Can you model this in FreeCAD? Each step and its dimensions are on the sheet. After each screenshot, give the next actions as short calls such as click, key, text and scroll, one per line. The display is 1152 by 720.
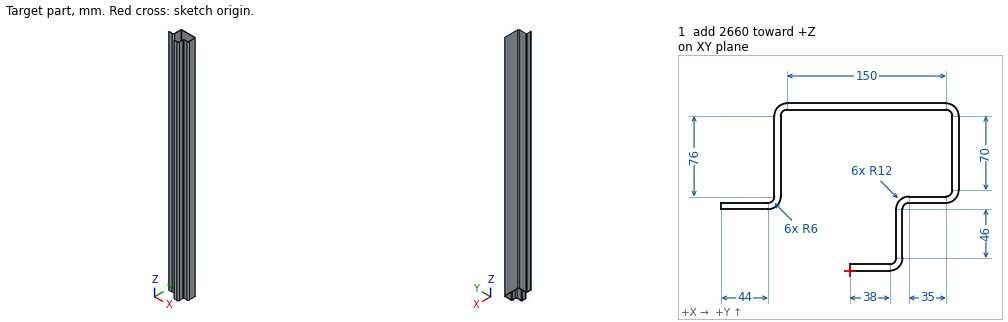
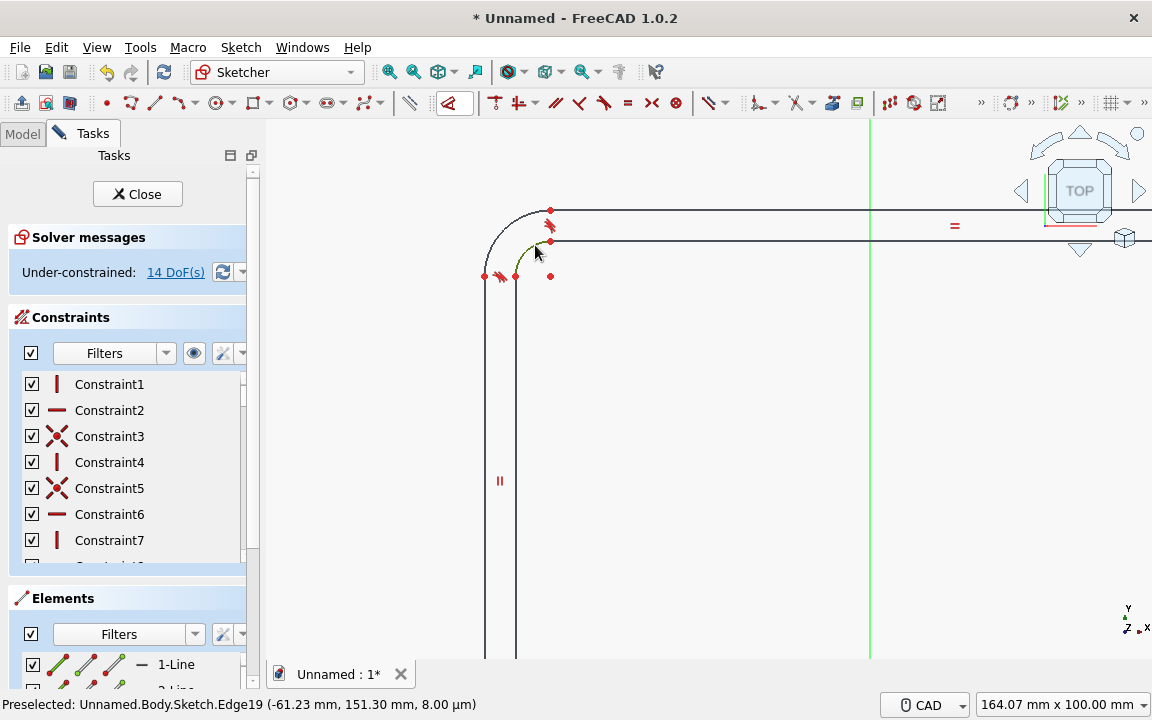
scroll(535, 246, down, 5)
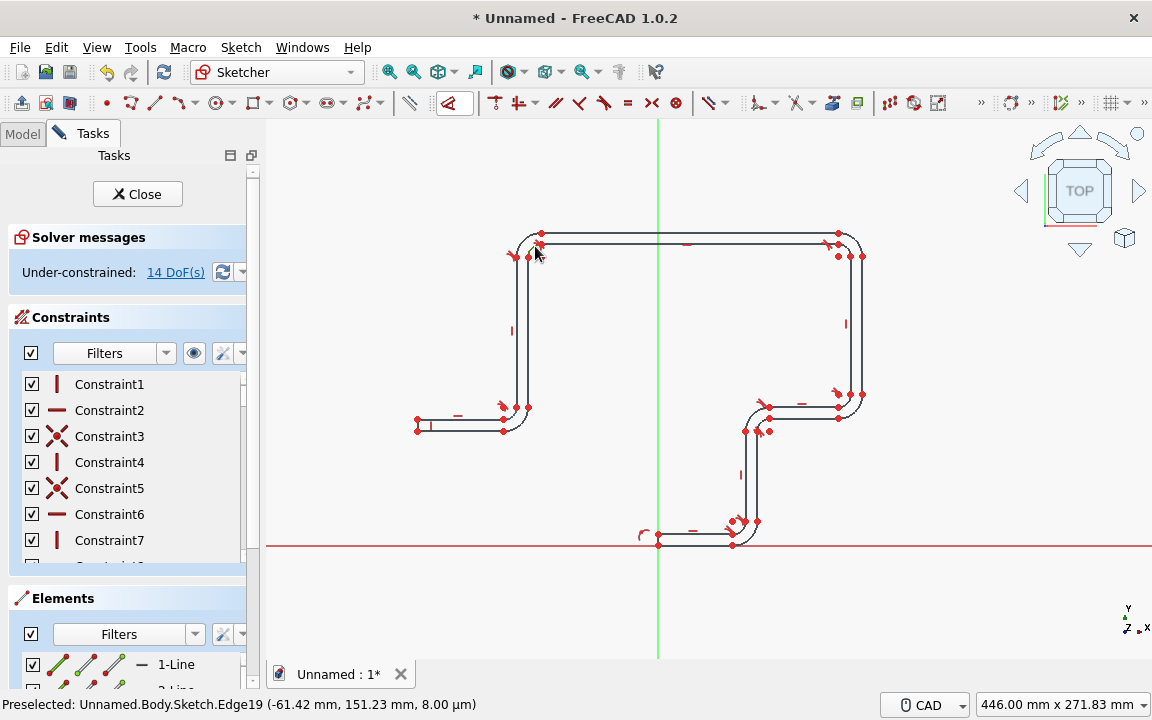
scroll(850, 251, up, 5)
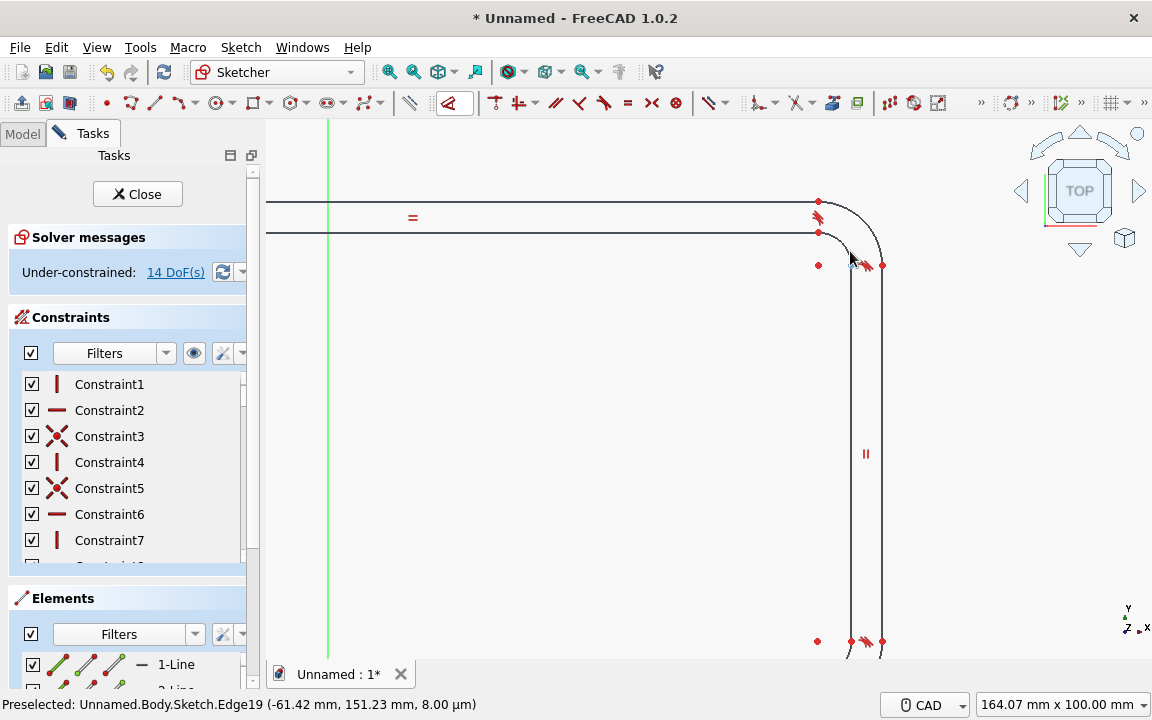
click(848, 251)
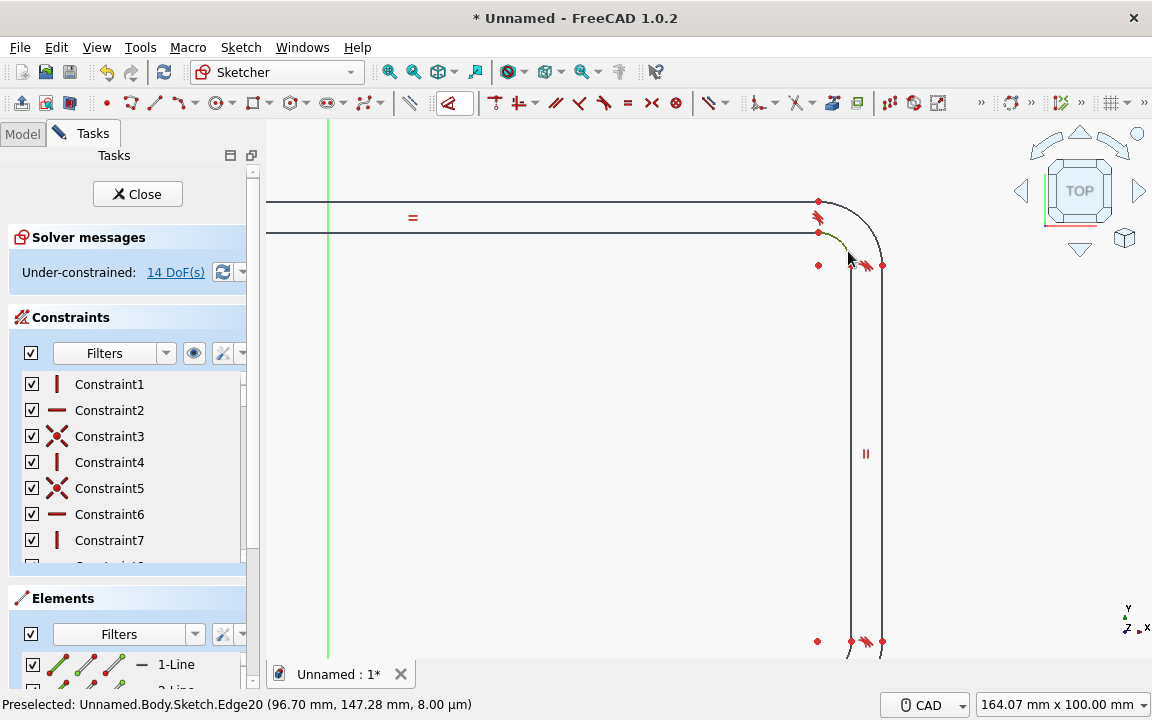
scroll(851, 251, down, 5)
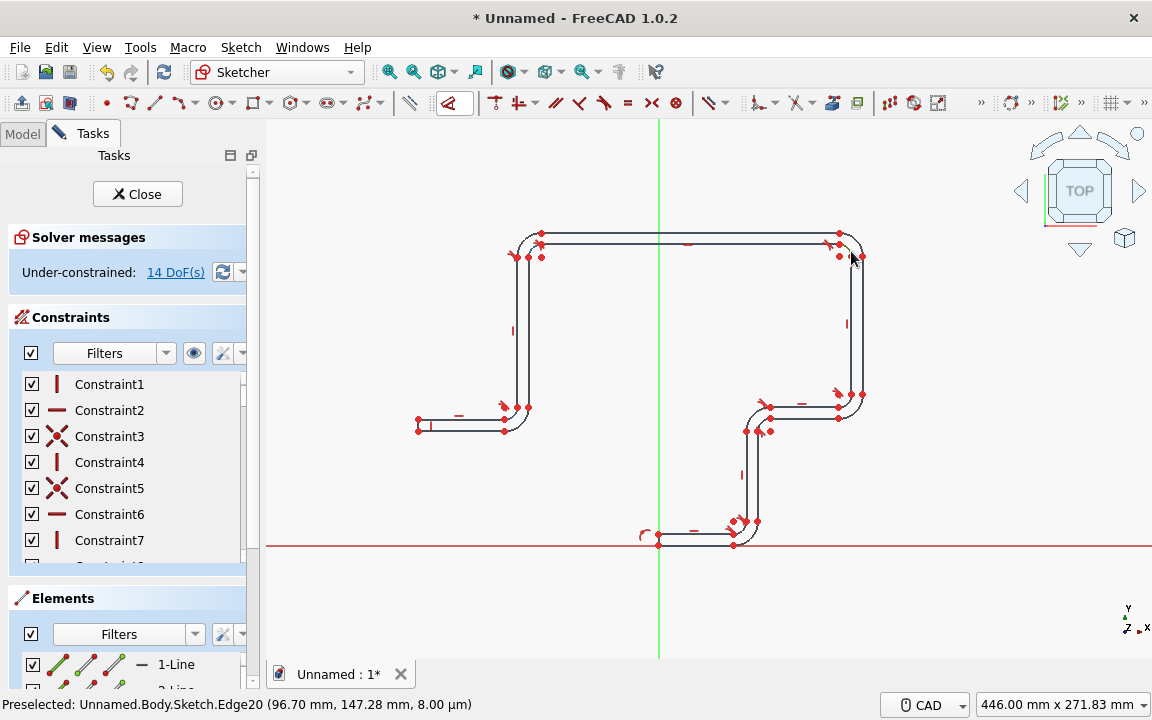
scroll(845, 406, up, 5)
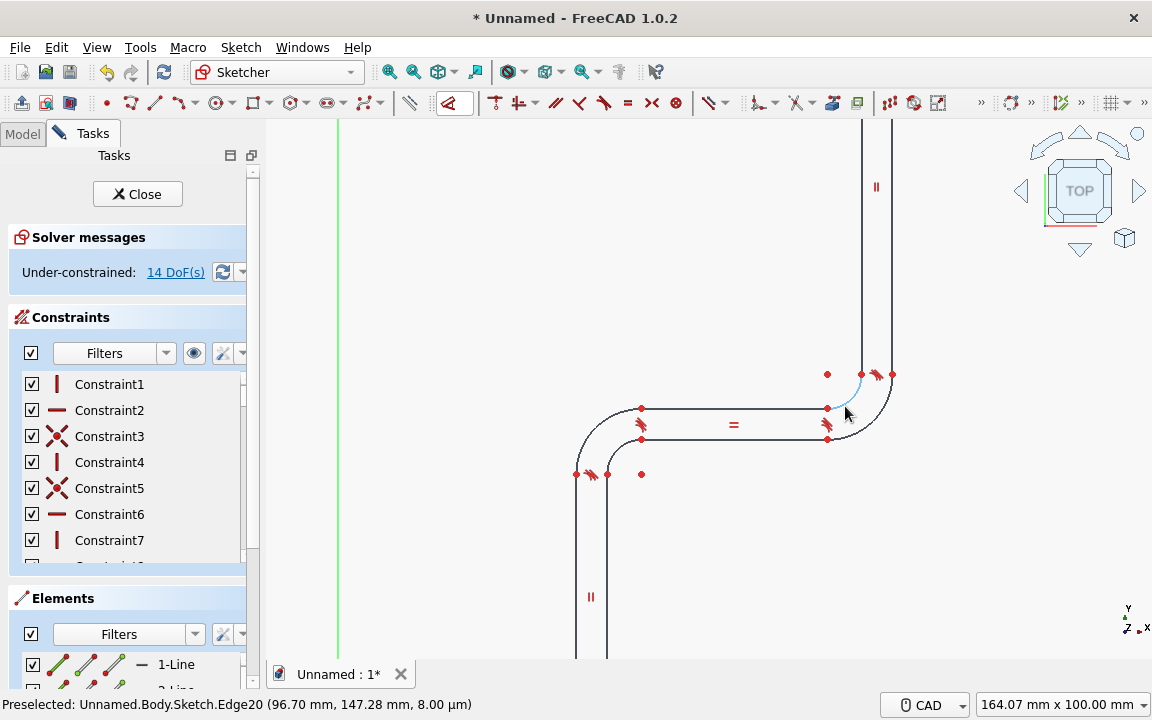
click(843, 405)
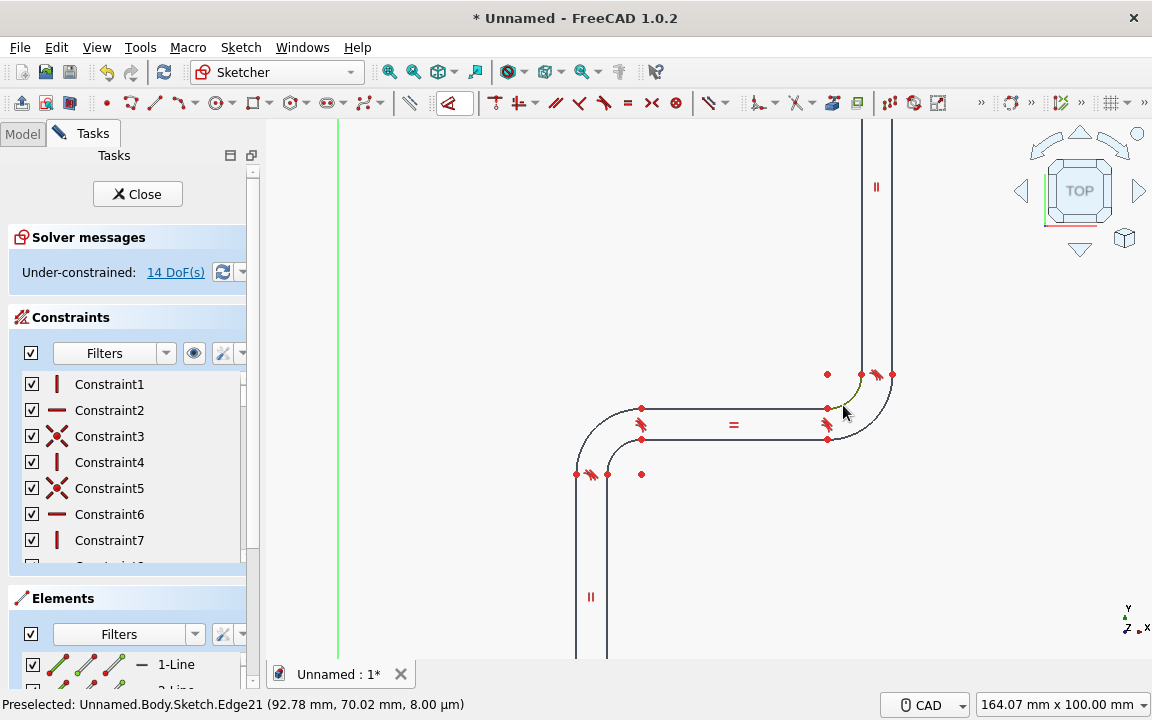
scroll(845, 407, down, 5)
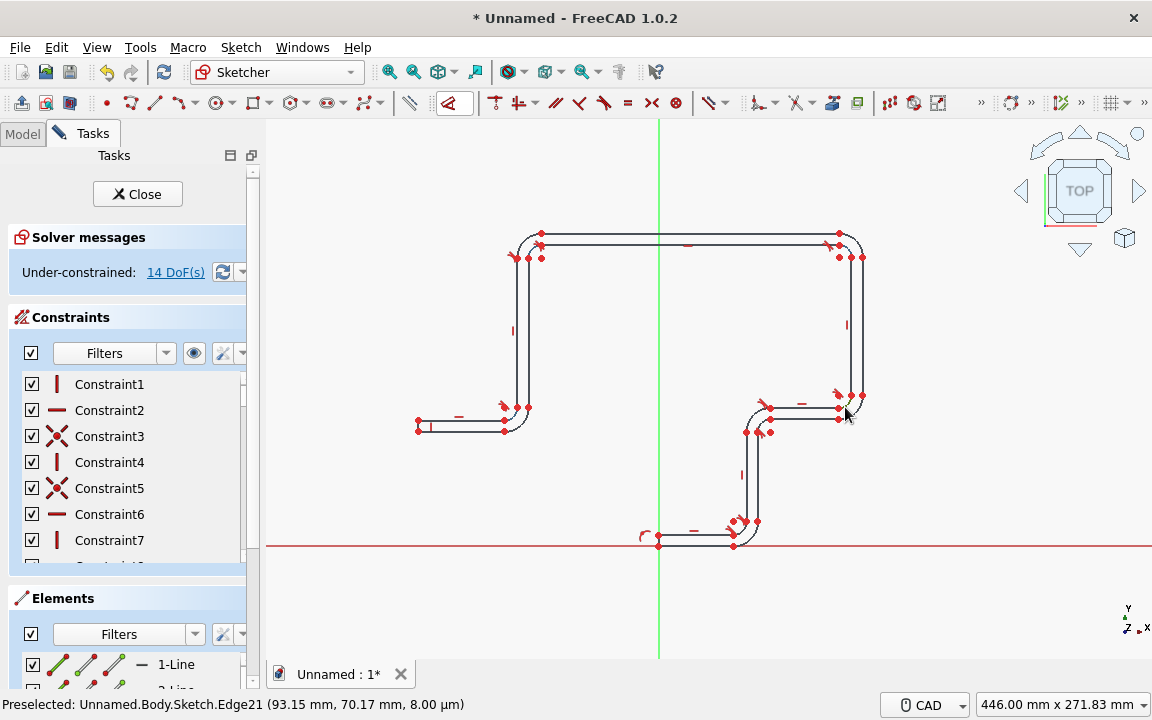
scroll(739, 534, up, 4)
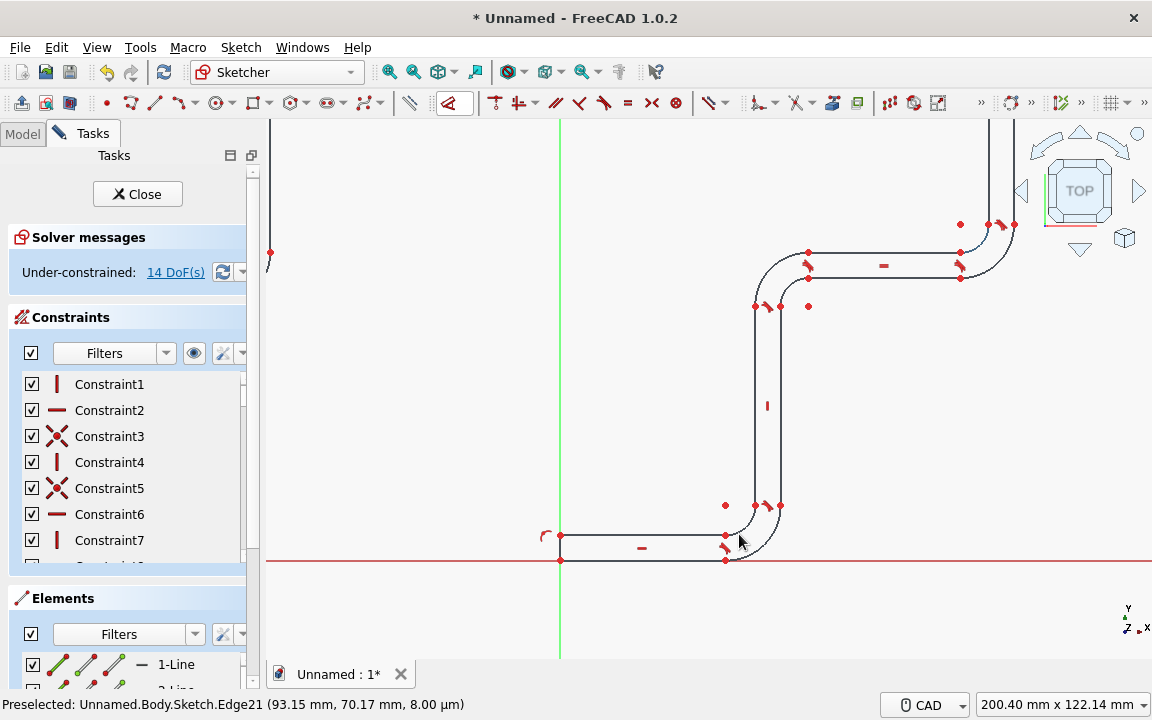
click(739, 532)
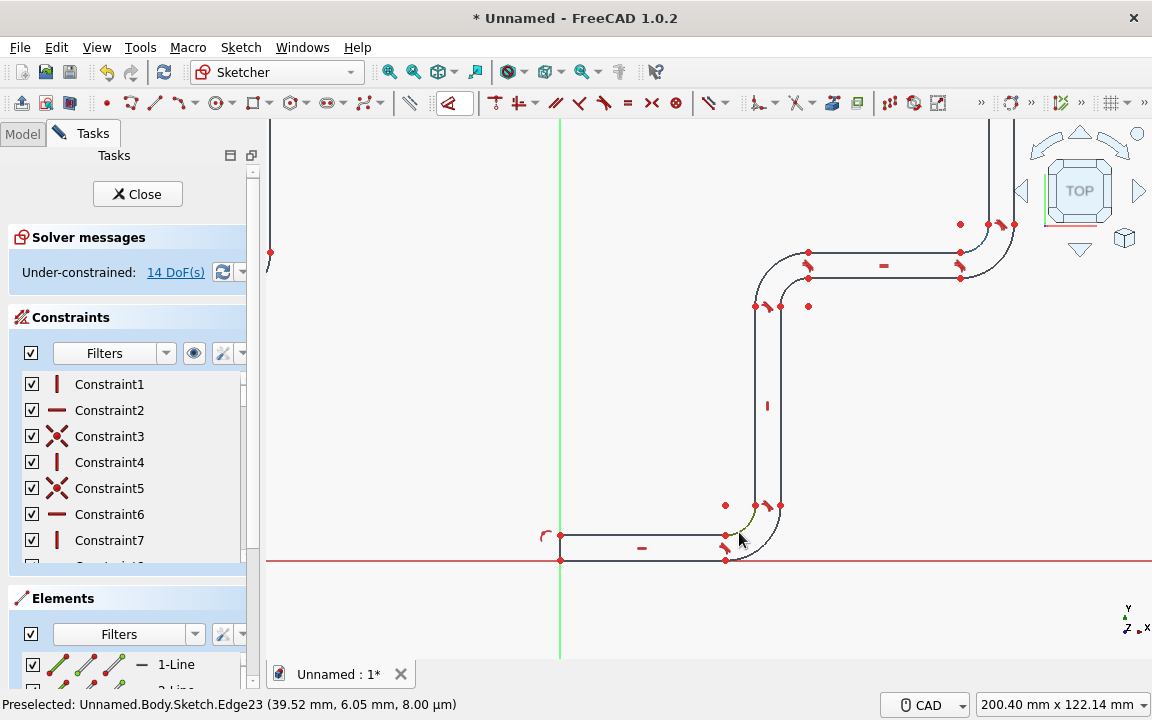
click(796, 281)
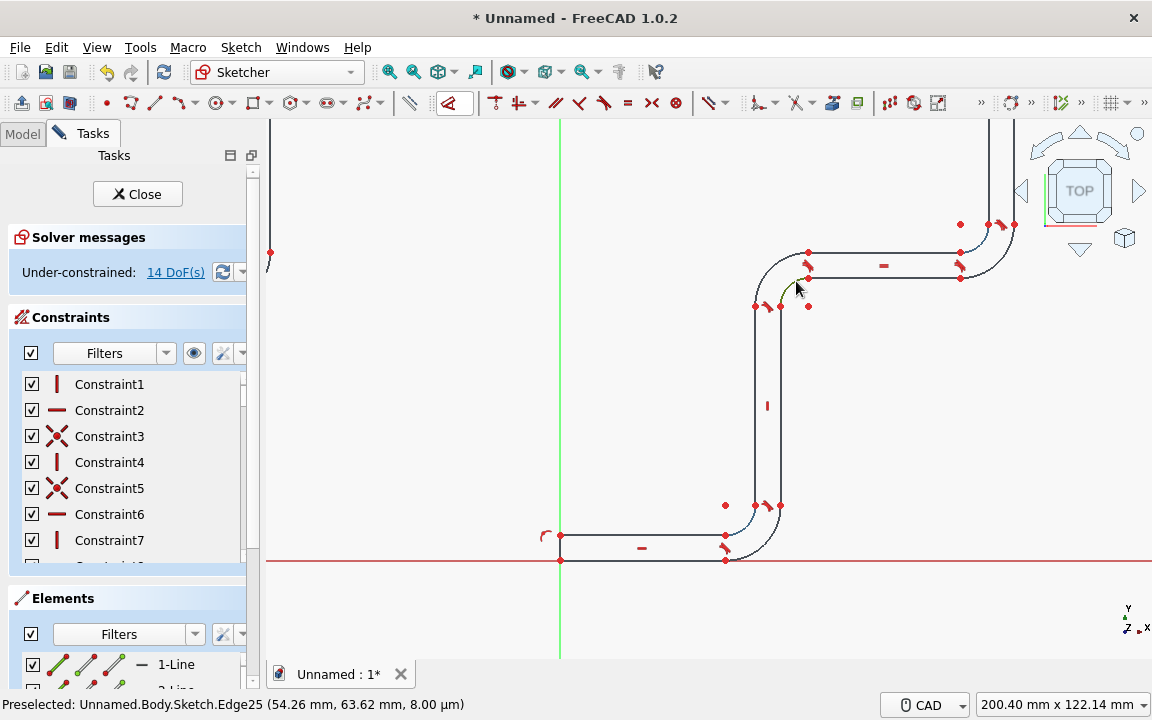
key(e)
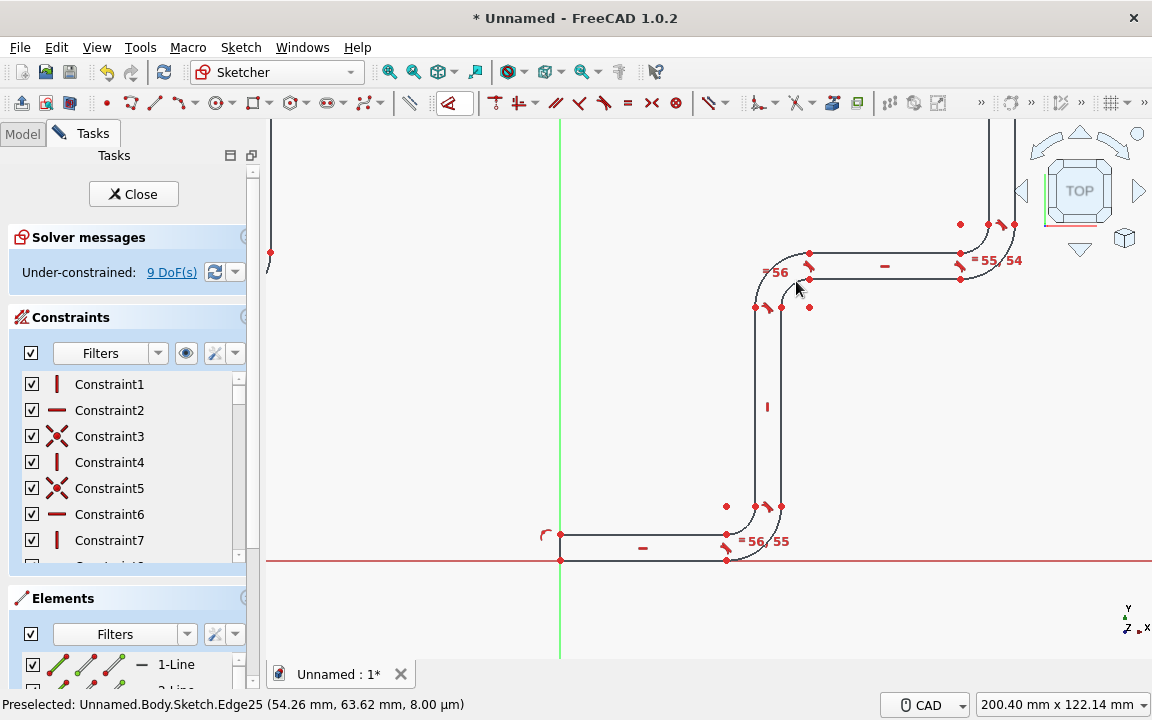
scroll(739, 534, down, 4)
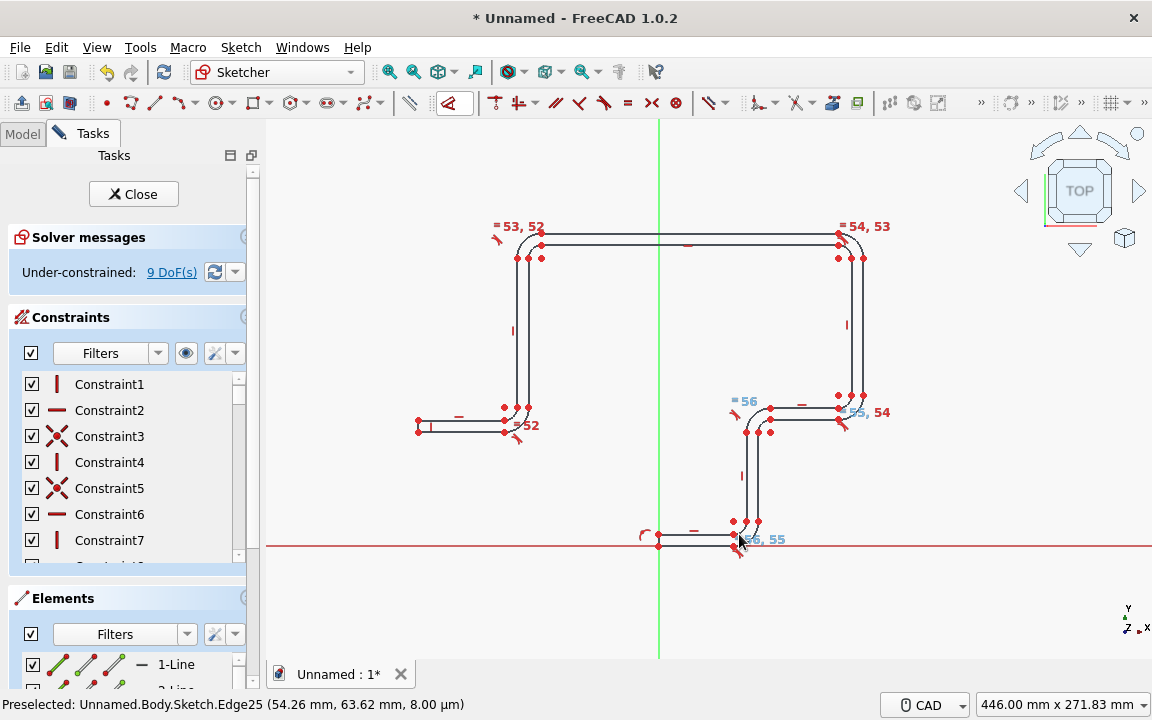
scroll(510, 419, up, 7)